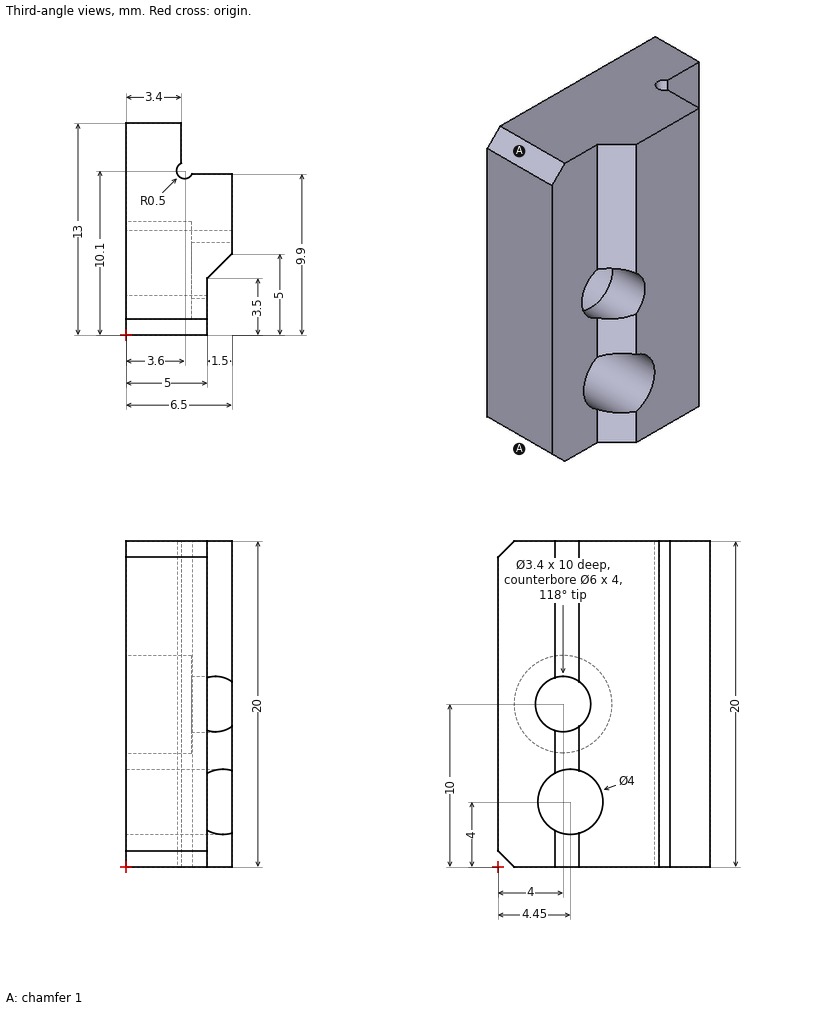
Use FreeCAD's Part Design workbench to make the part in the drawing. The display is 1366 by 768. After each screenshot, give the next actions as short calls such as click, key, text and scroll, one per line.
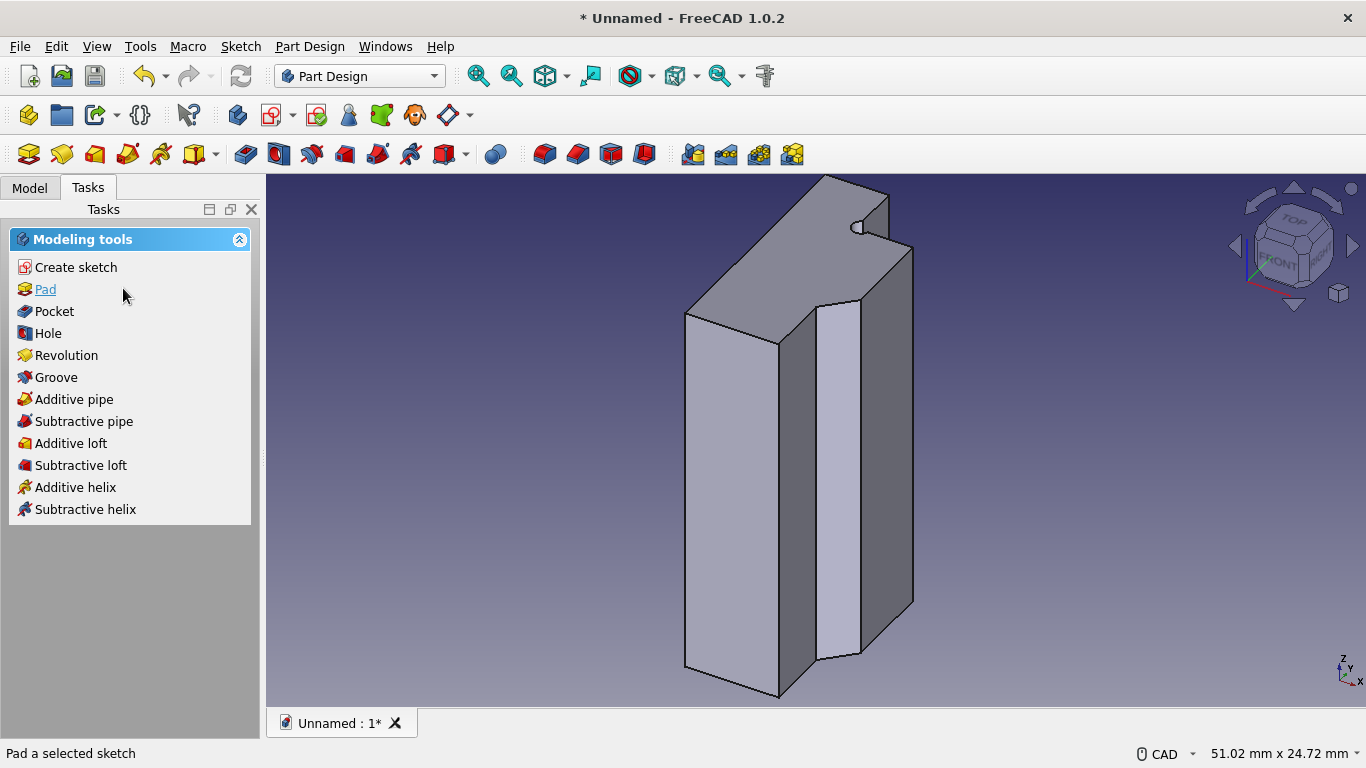
click(279, 154)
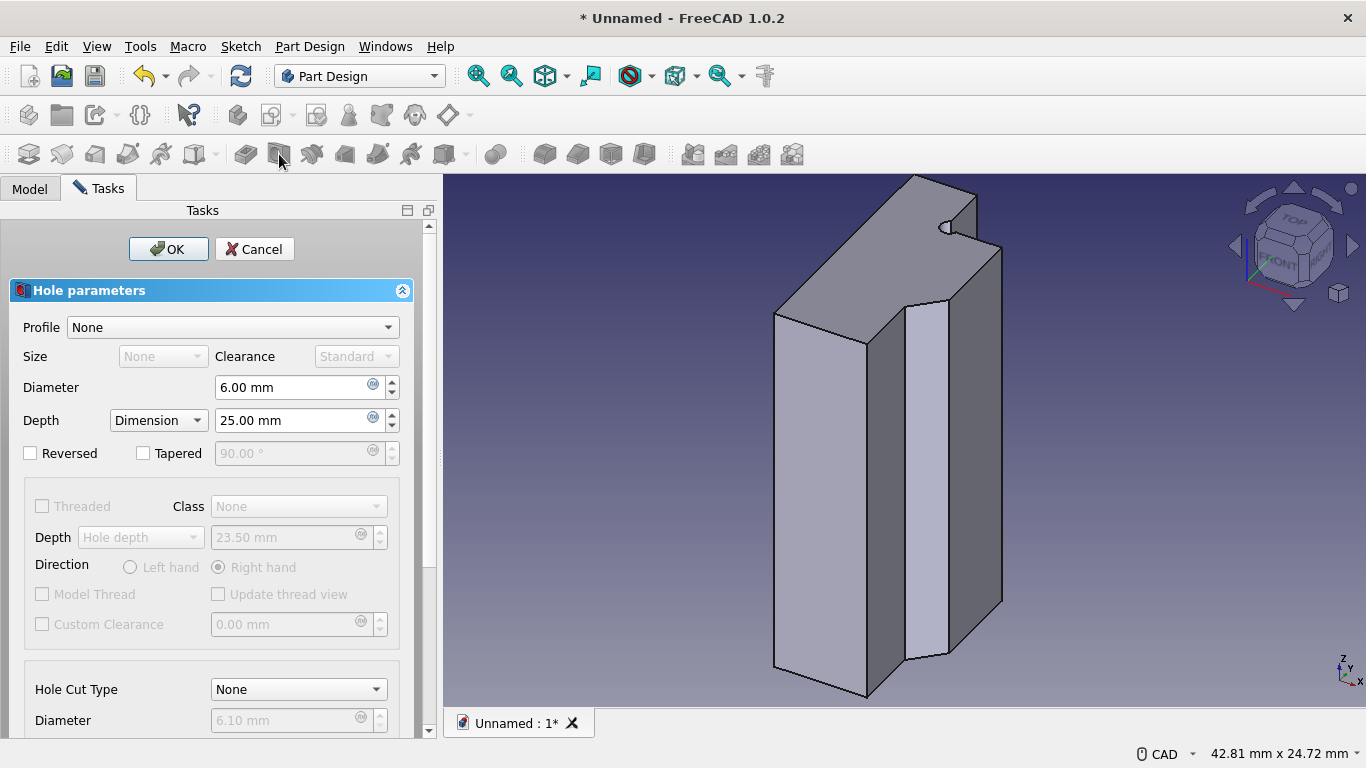
triple_click(300, 388)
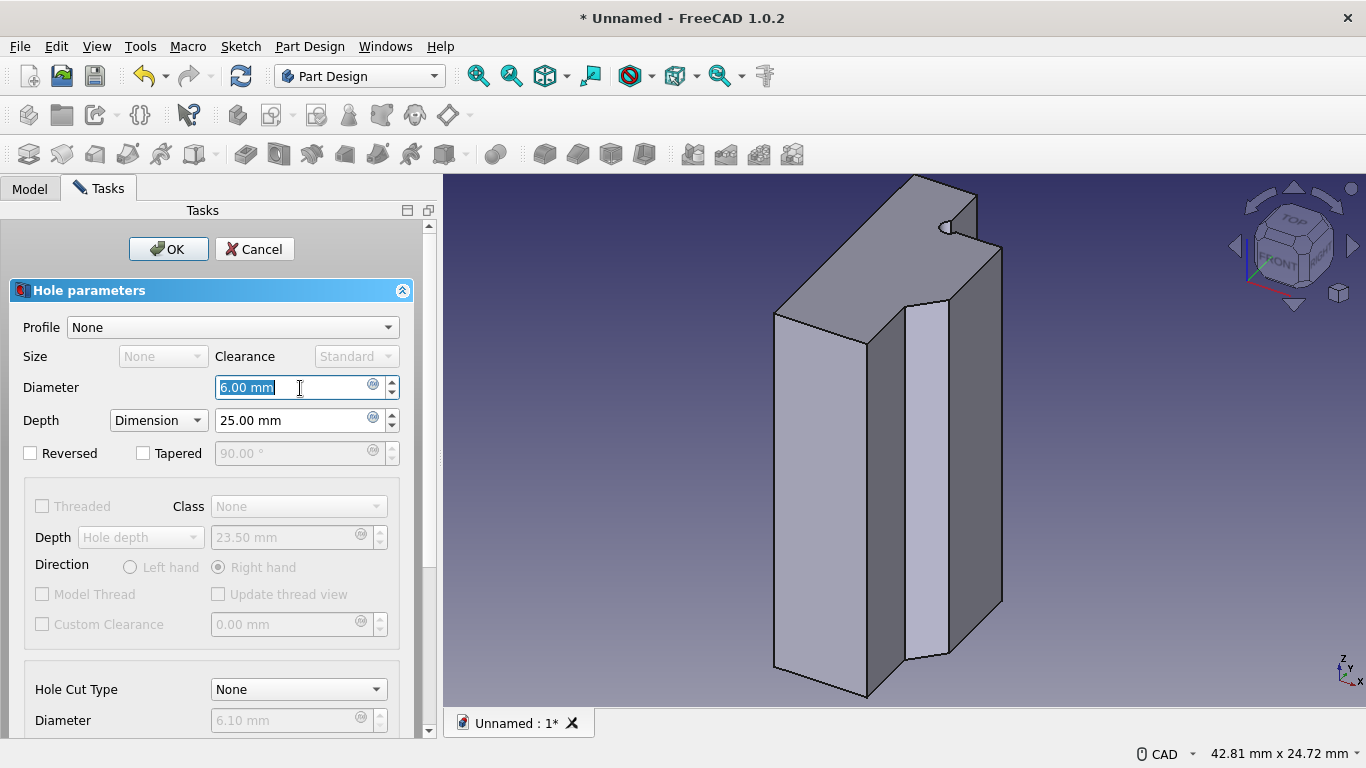
text(3.4)
key(Tab)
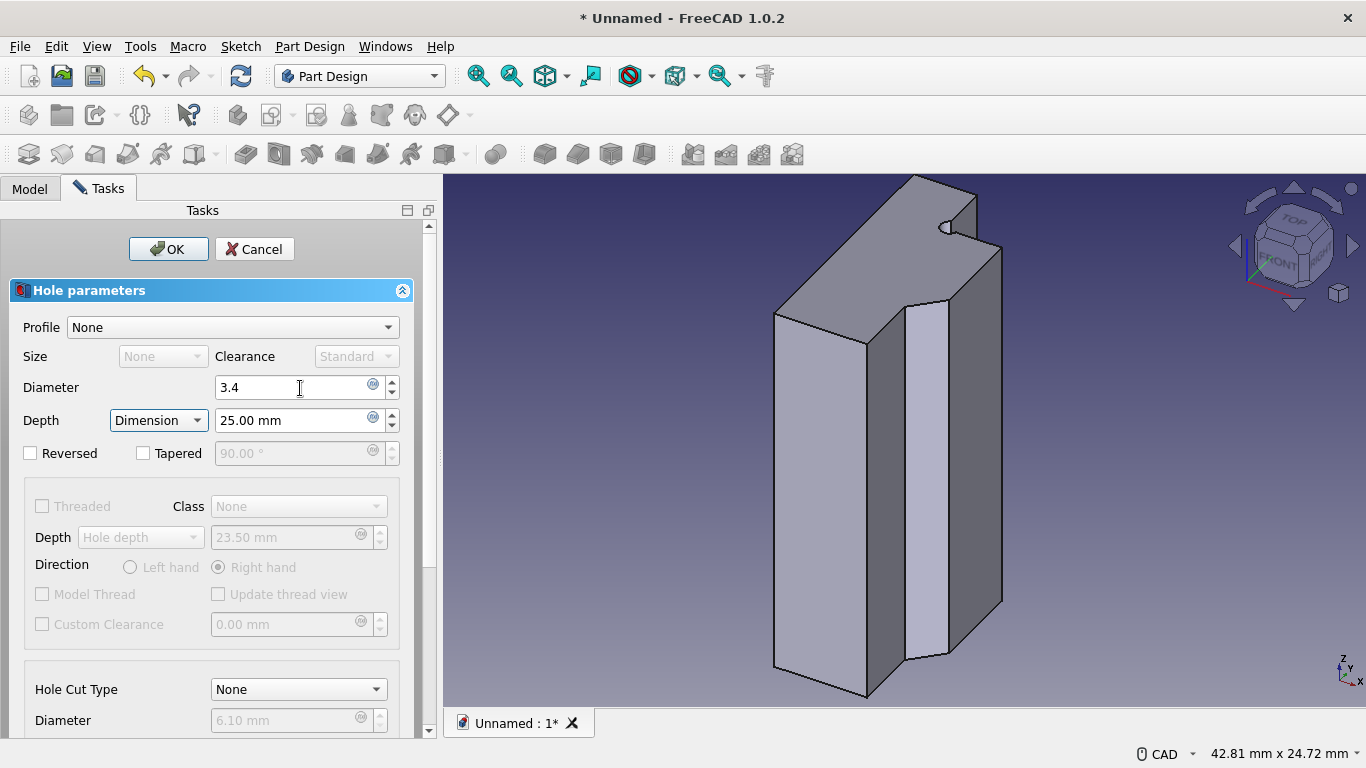
triple_click(300, 420)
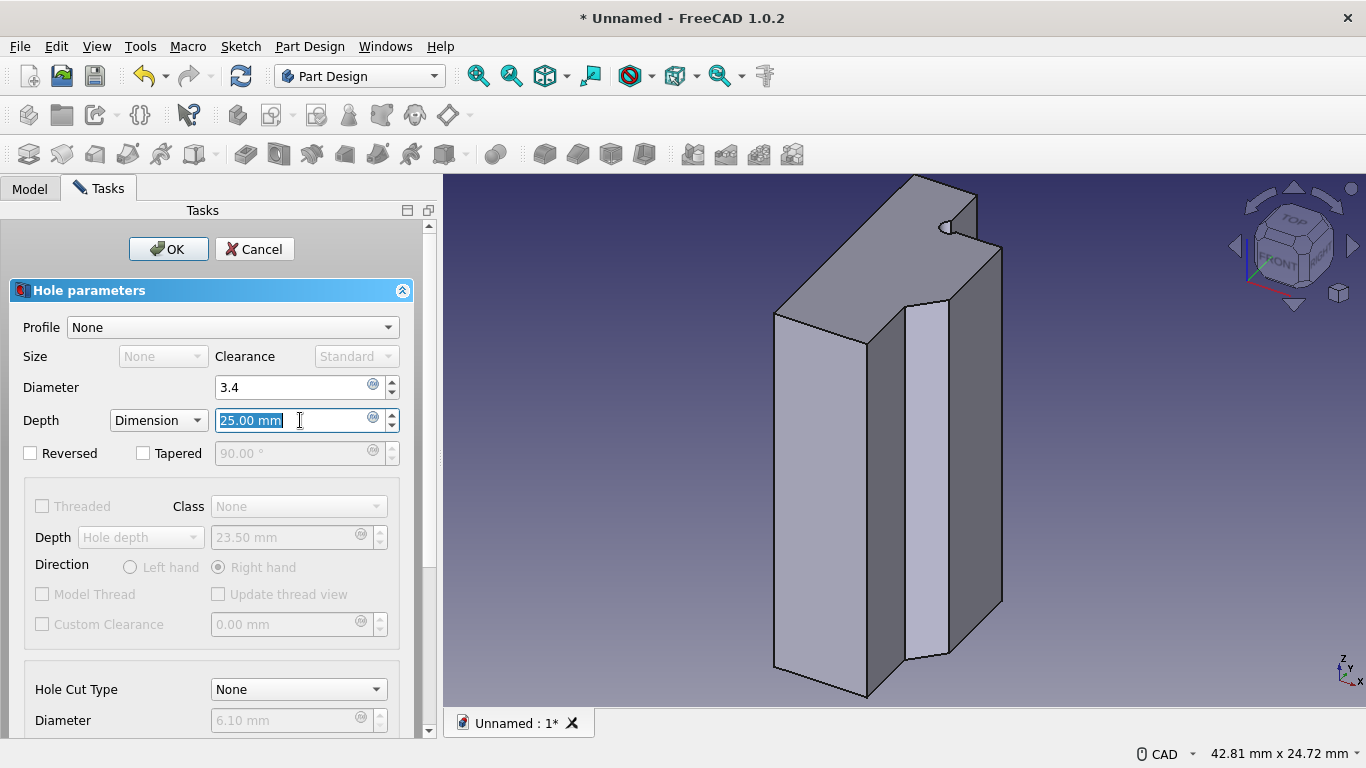
text(10)
key(Tab)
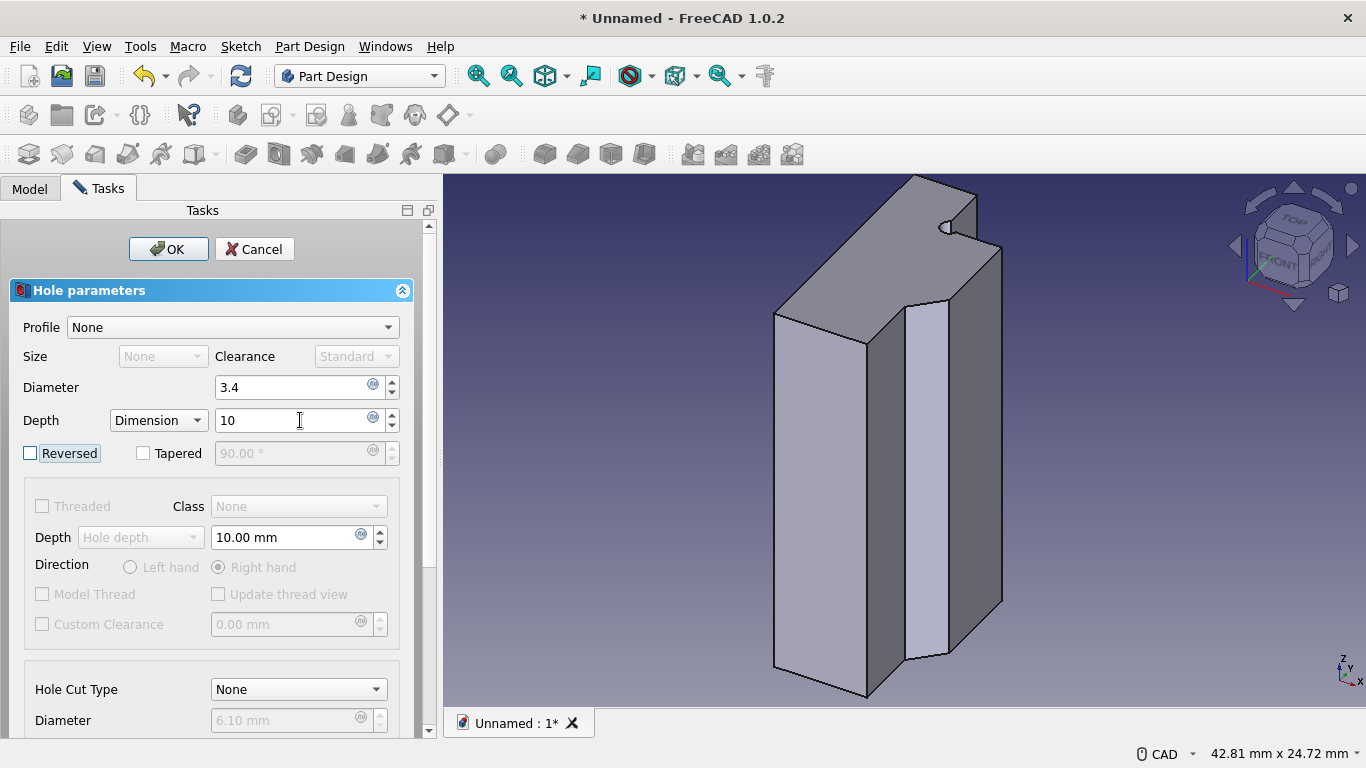
click(31, 453)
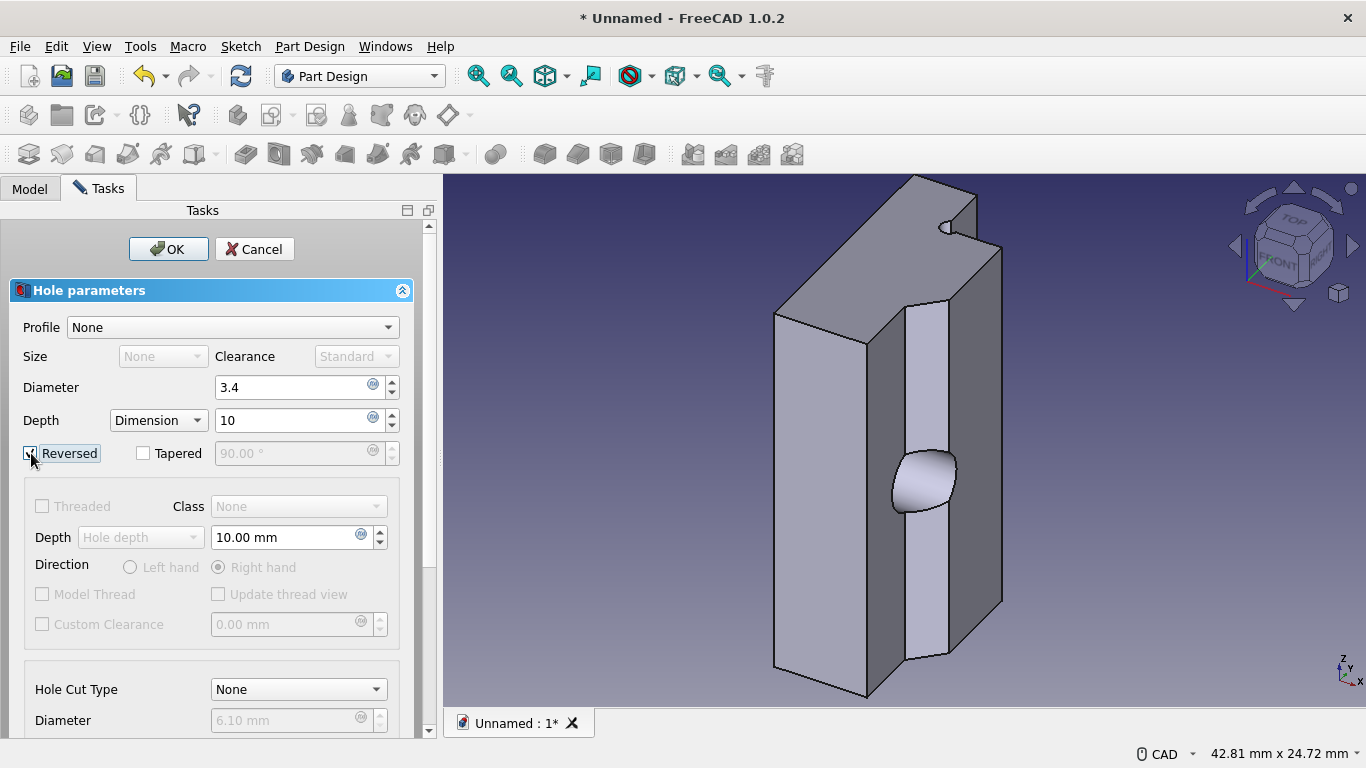
click(300, 690)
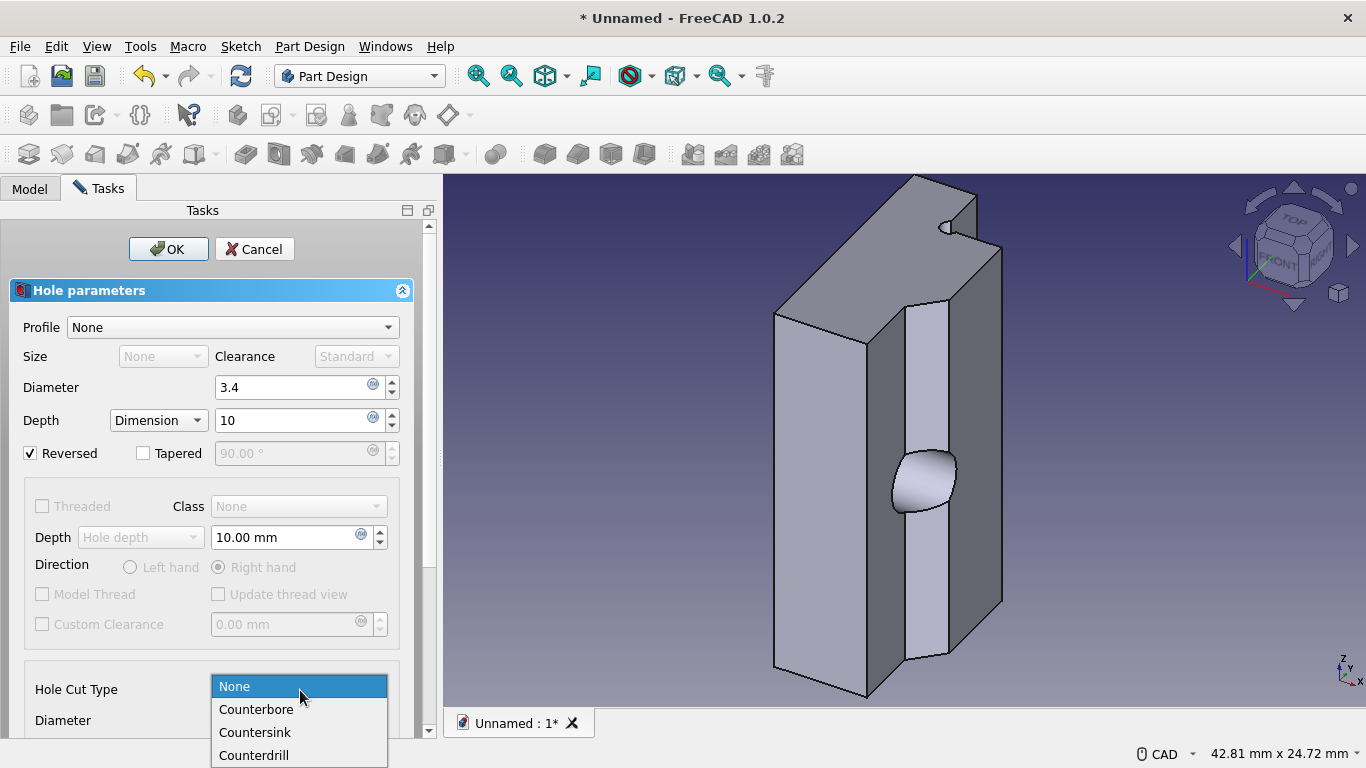
click(298, 710)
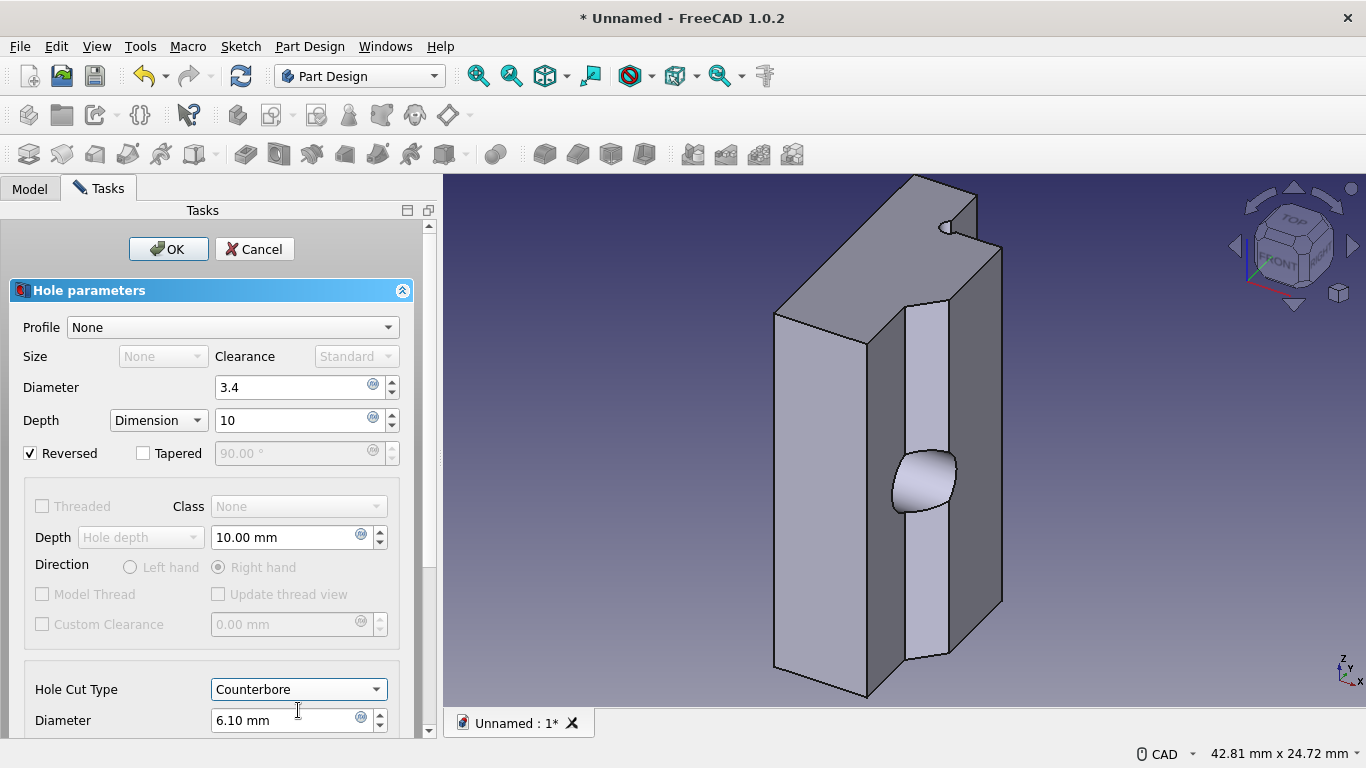
triple_click(292, 720)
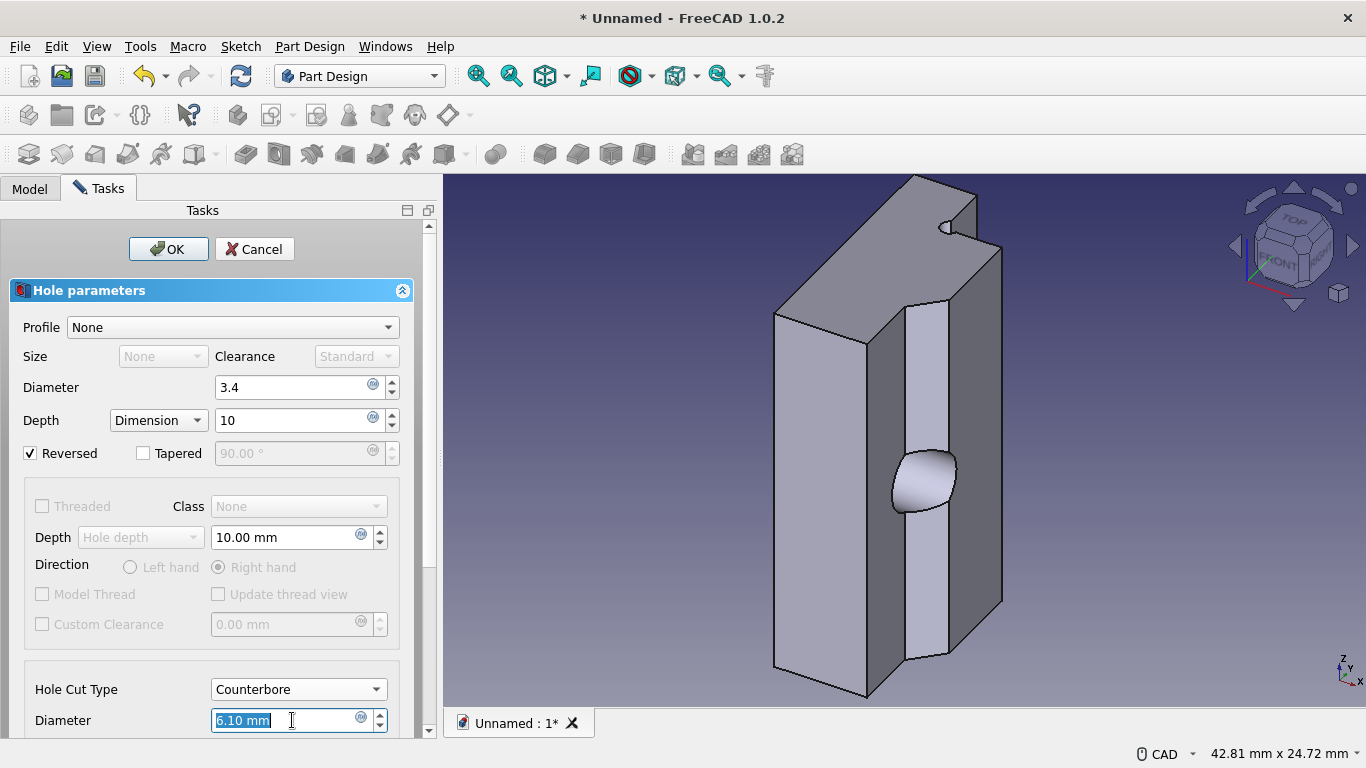
text(6)
key(Tab)